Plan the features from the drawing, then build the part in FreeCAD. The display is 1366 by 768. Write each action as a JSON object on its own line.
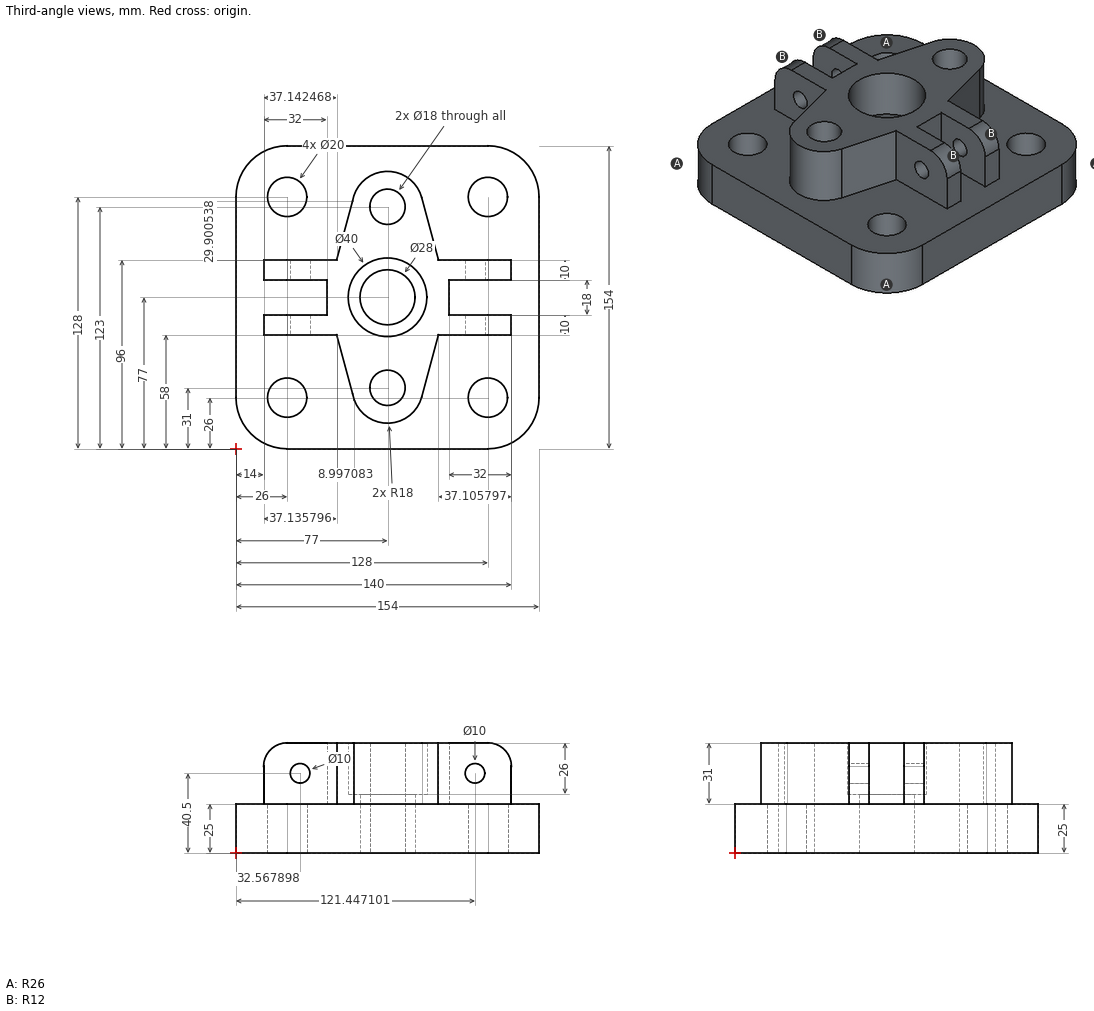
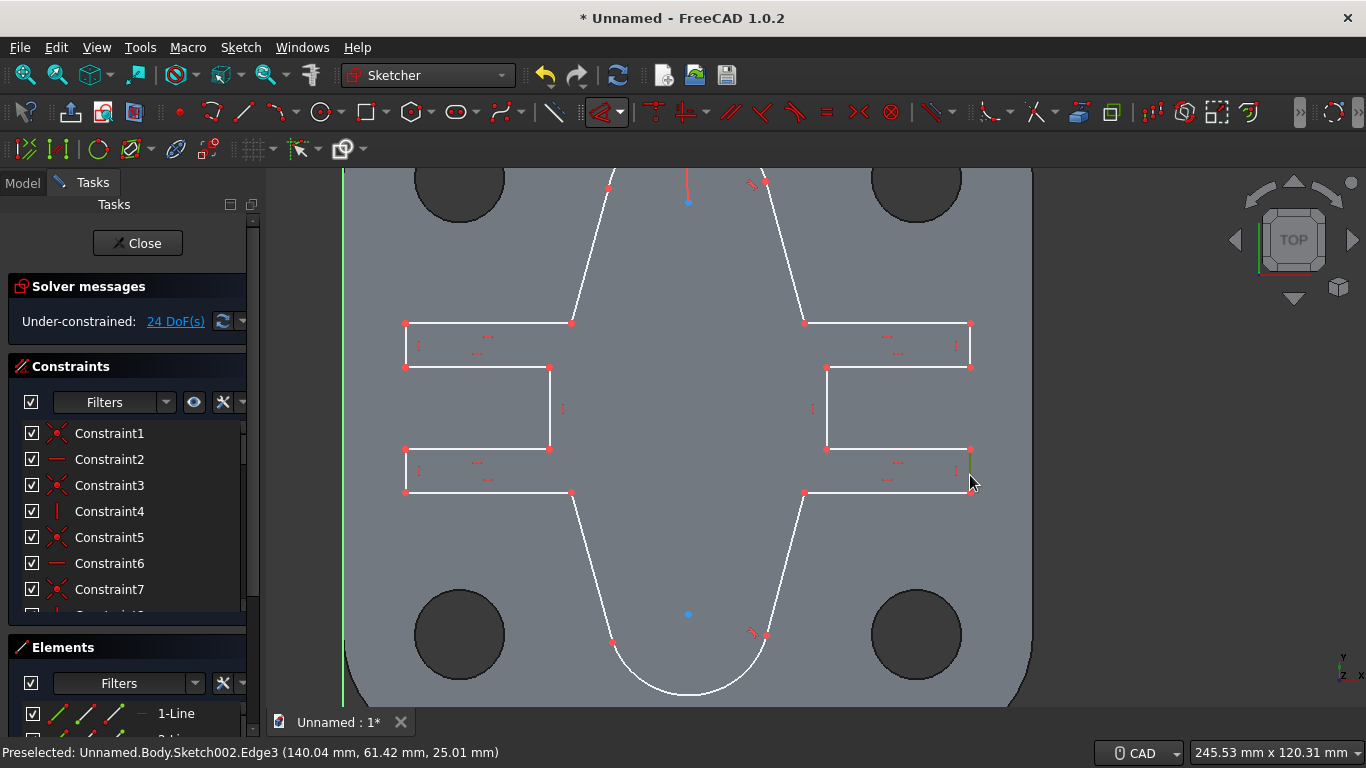
{"action": "key", "text": "i"}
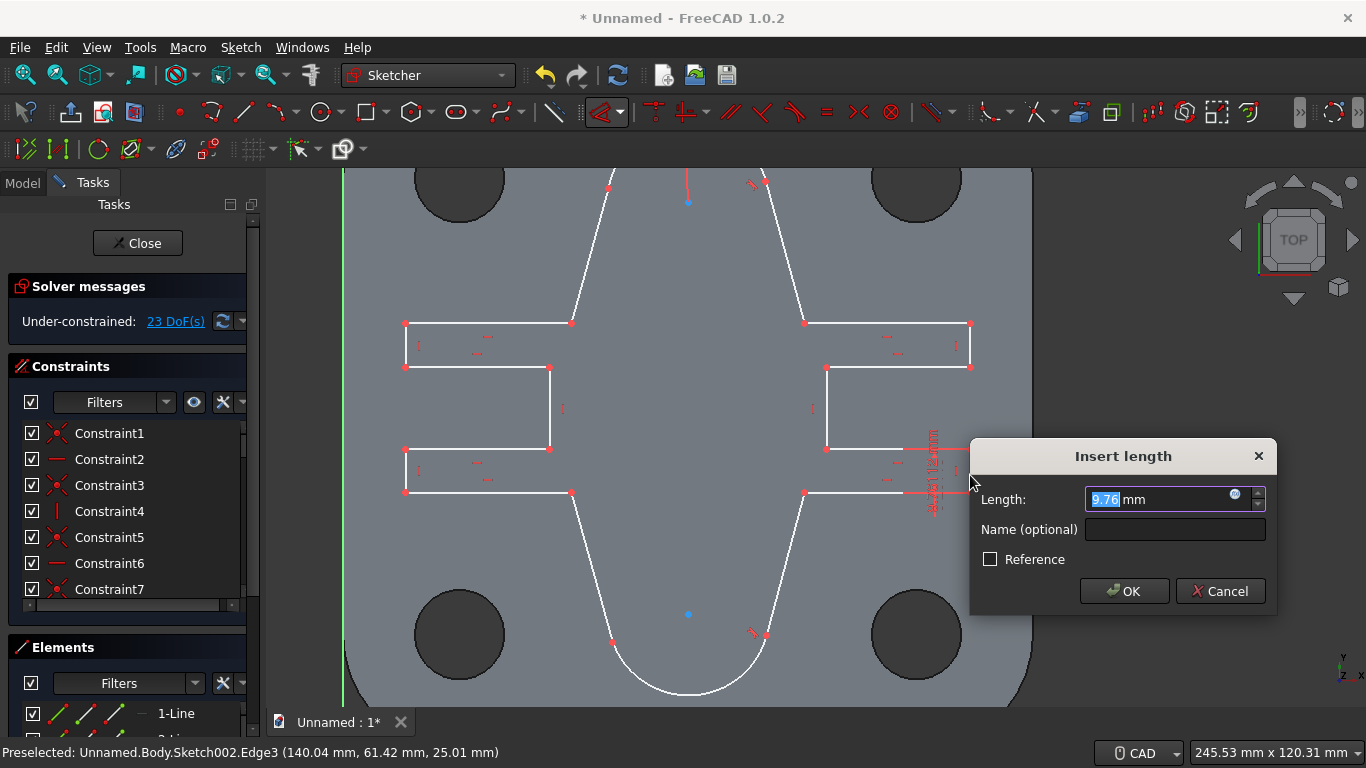
{"action": "type", "text": "10"}
{"action": "key", "text": "Return"}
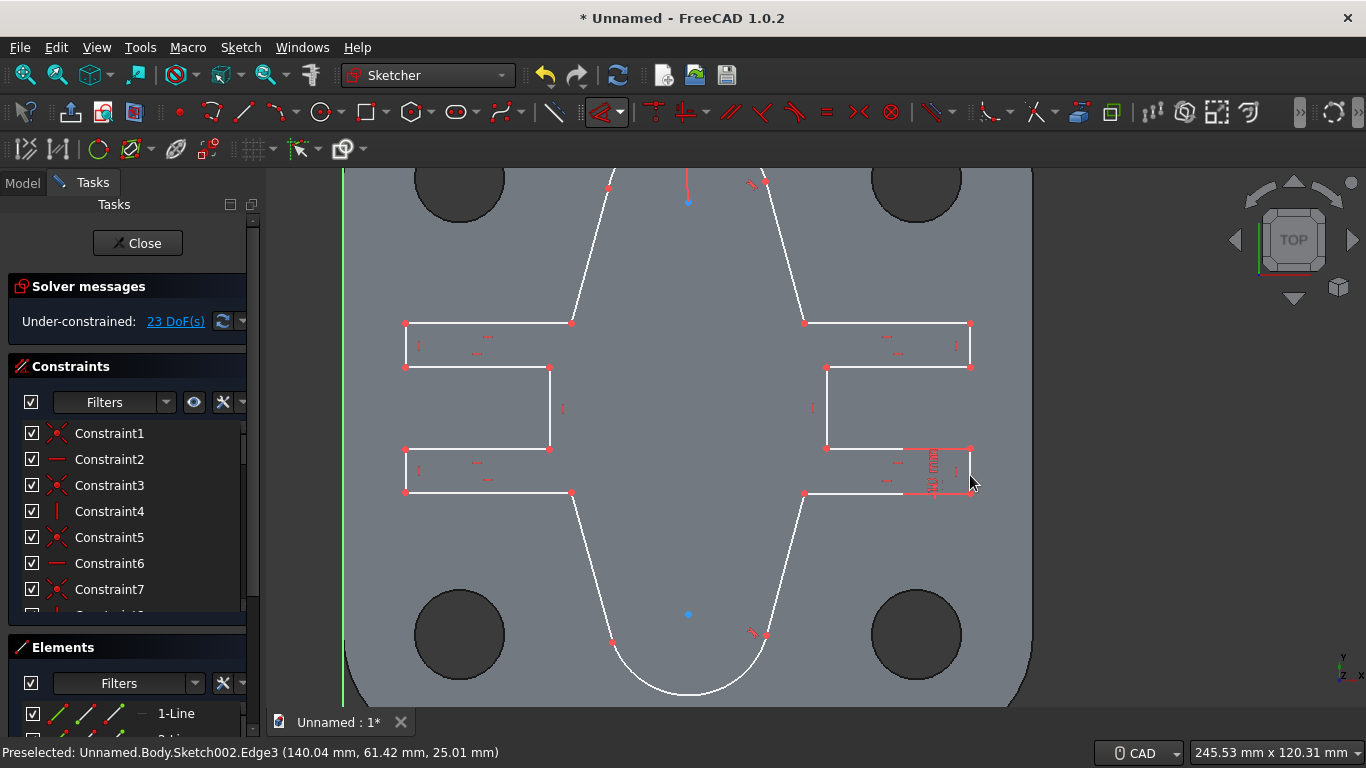
{"action": "left_click", "coordinate": [870, 449]}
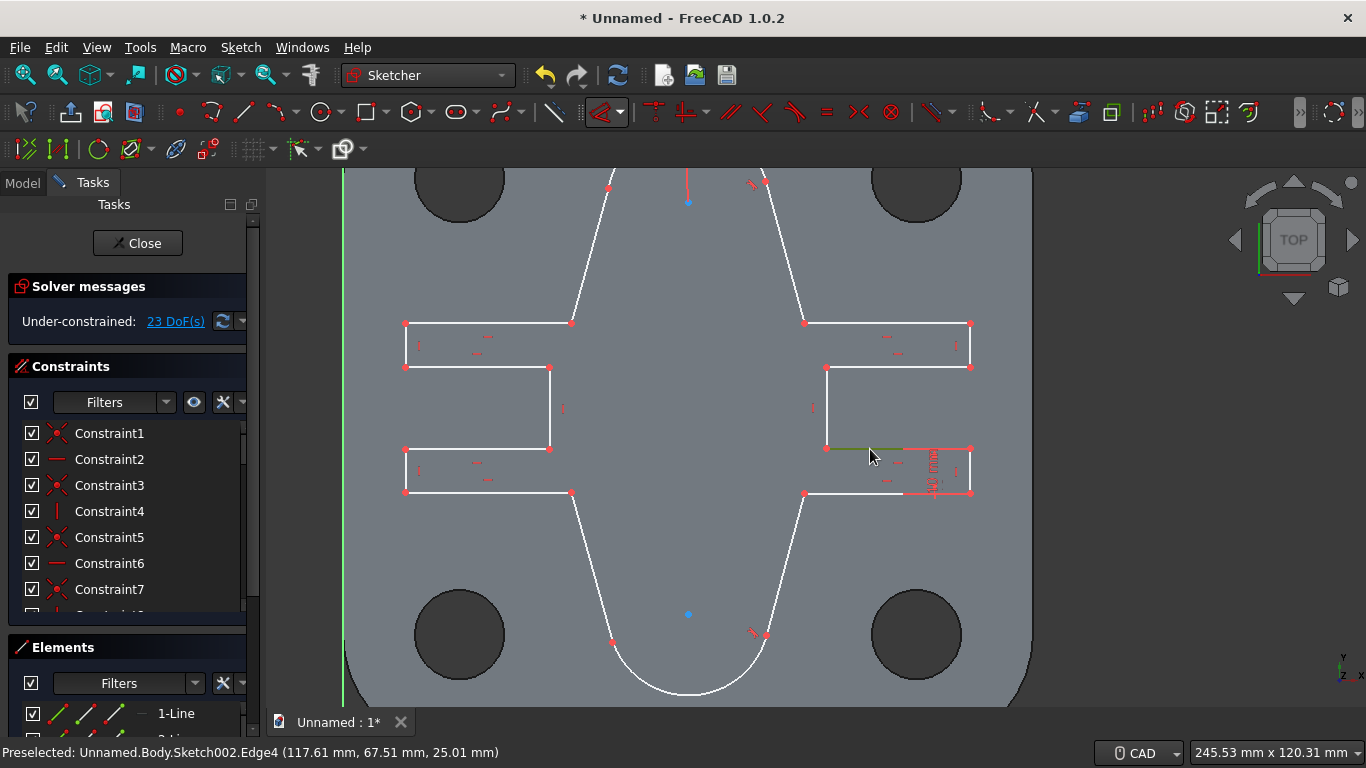
{"action": "left_click", "coordinate": [622, 112]}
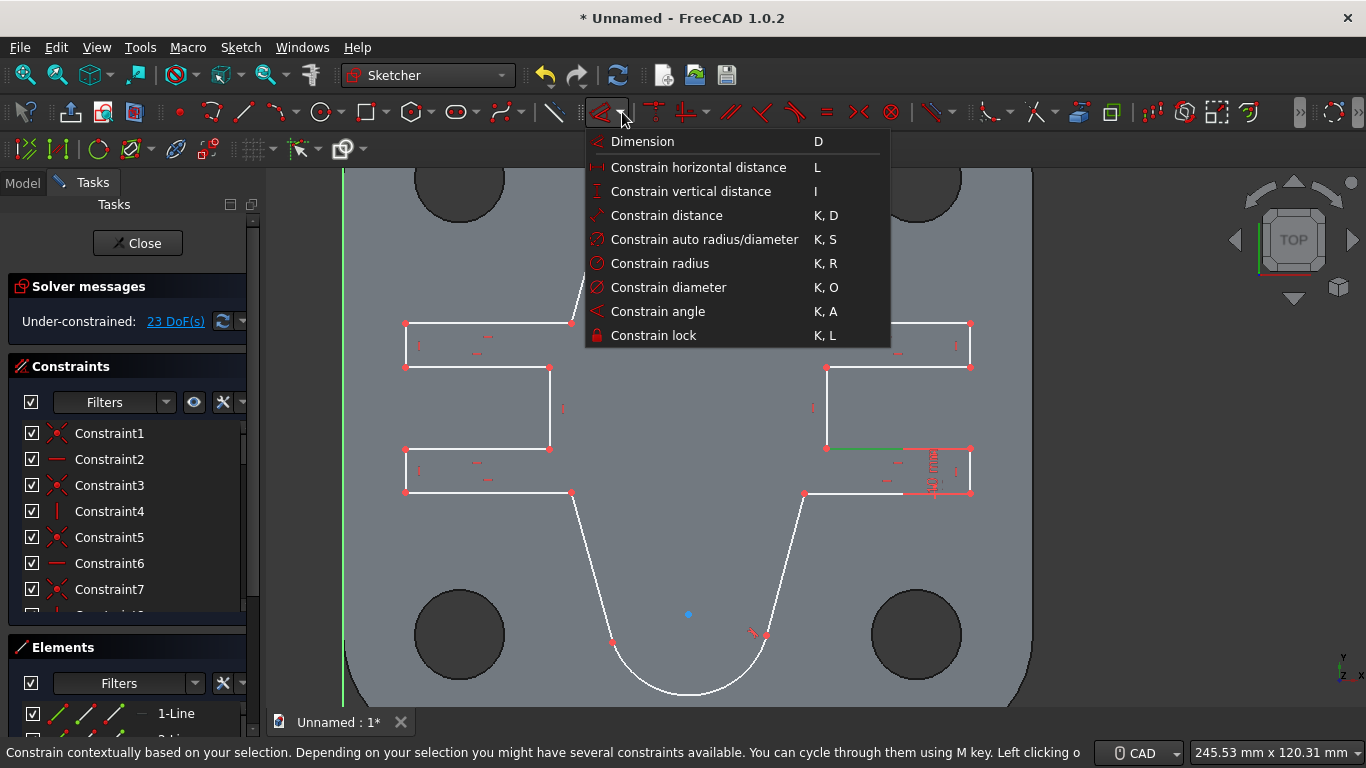
{"action": "left_click", "coordinate": [738, 167]}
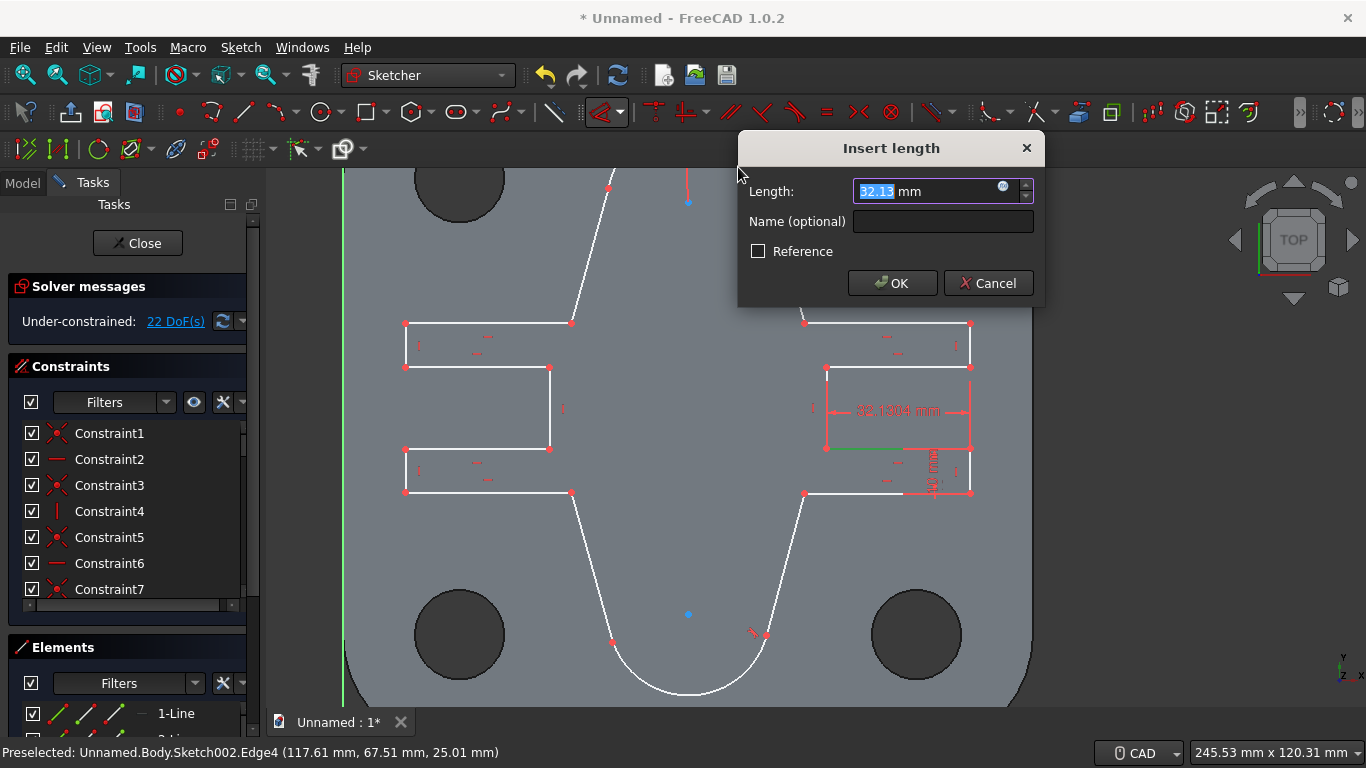
{"action": "type", "text": "32"}
{"action": "key", "text": "Return"}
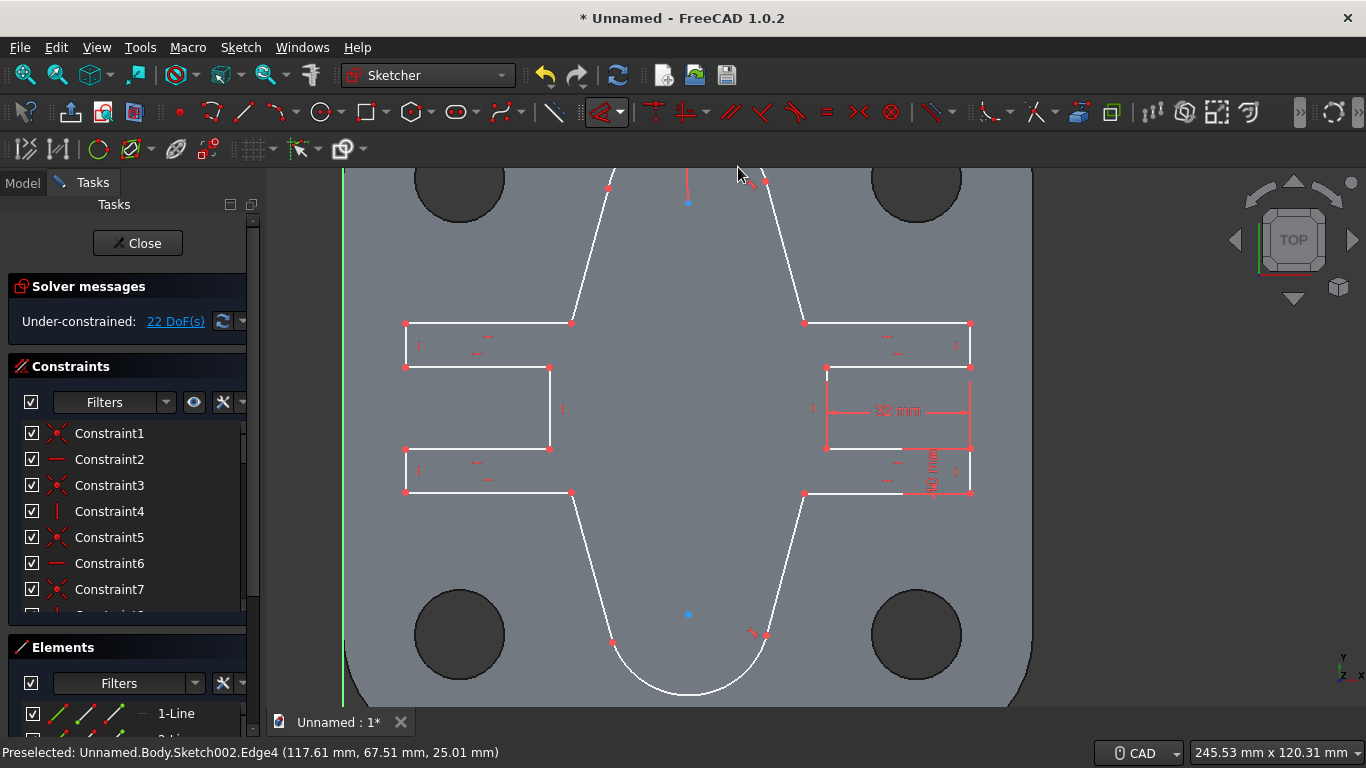
{"action": "left_click", "coordinate": [827, 424]}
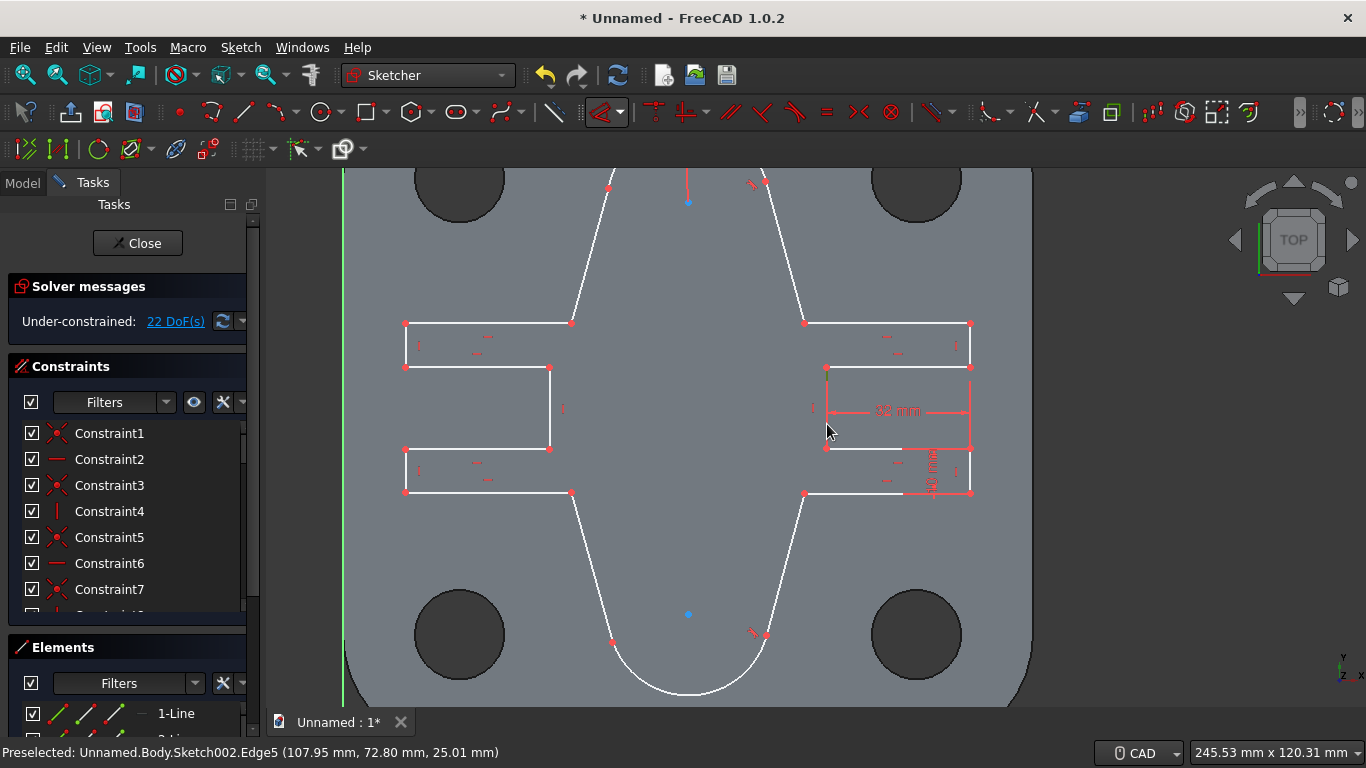
{"action": "key", "text": "i"}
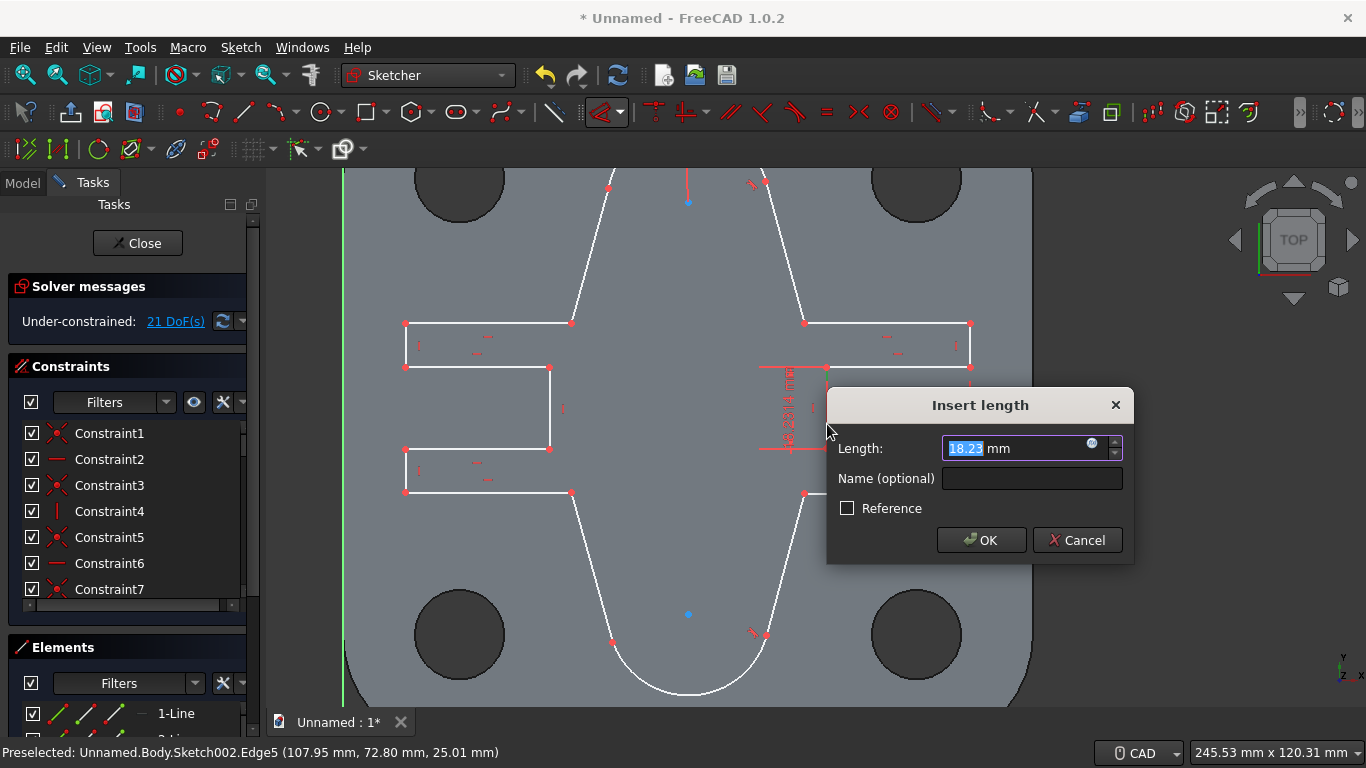
{"action": "type", "text": "18"}
{"action": "key", "text": "Return"}